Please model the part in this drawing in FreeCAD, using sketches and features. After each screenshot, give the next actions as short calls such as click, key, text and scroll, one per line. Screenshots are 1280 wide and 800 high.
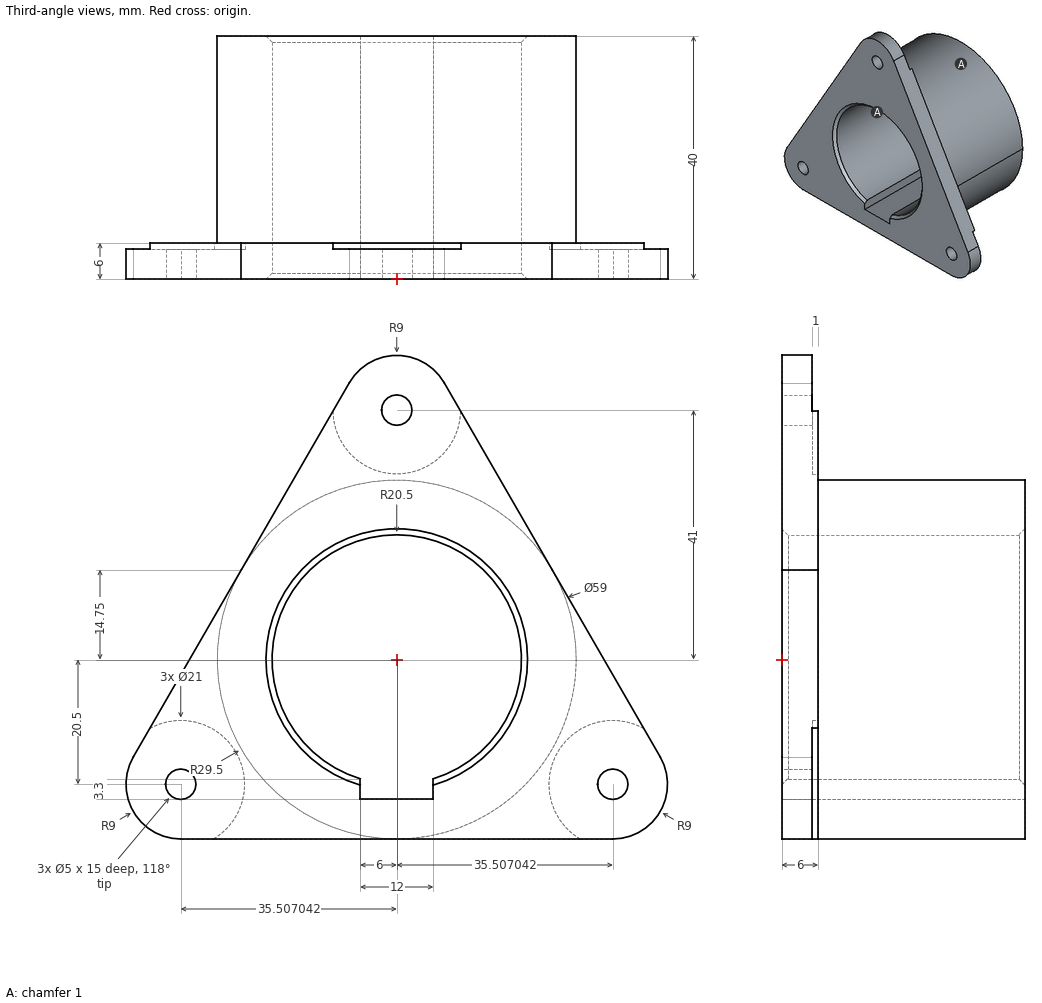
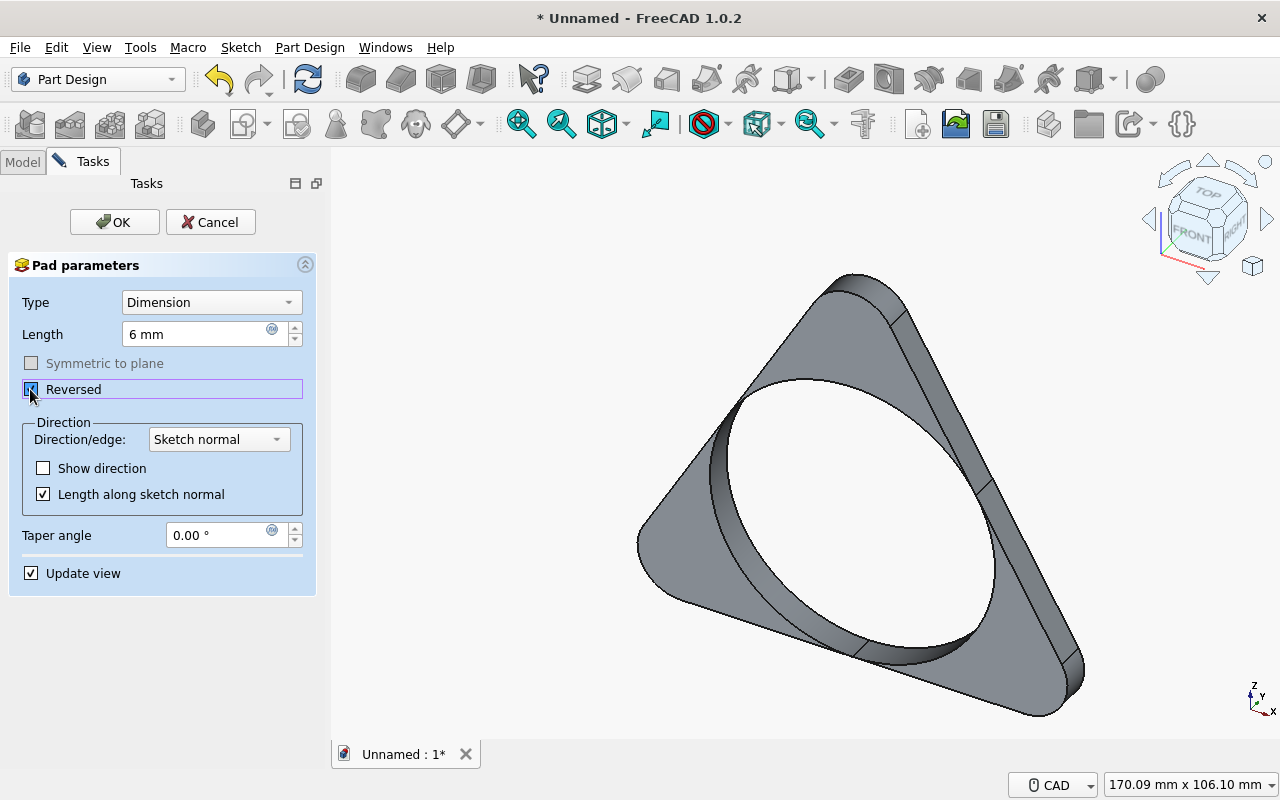
click(115, 222)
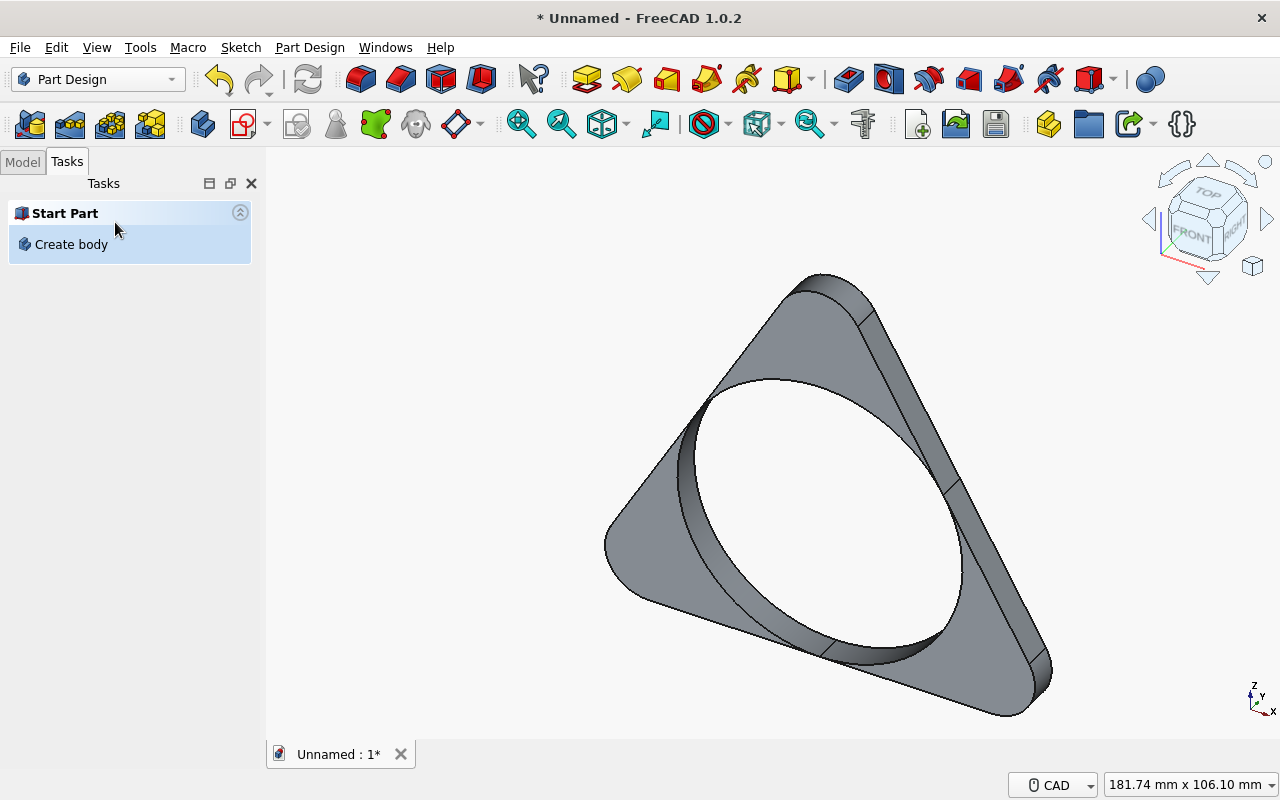
click(23, 161)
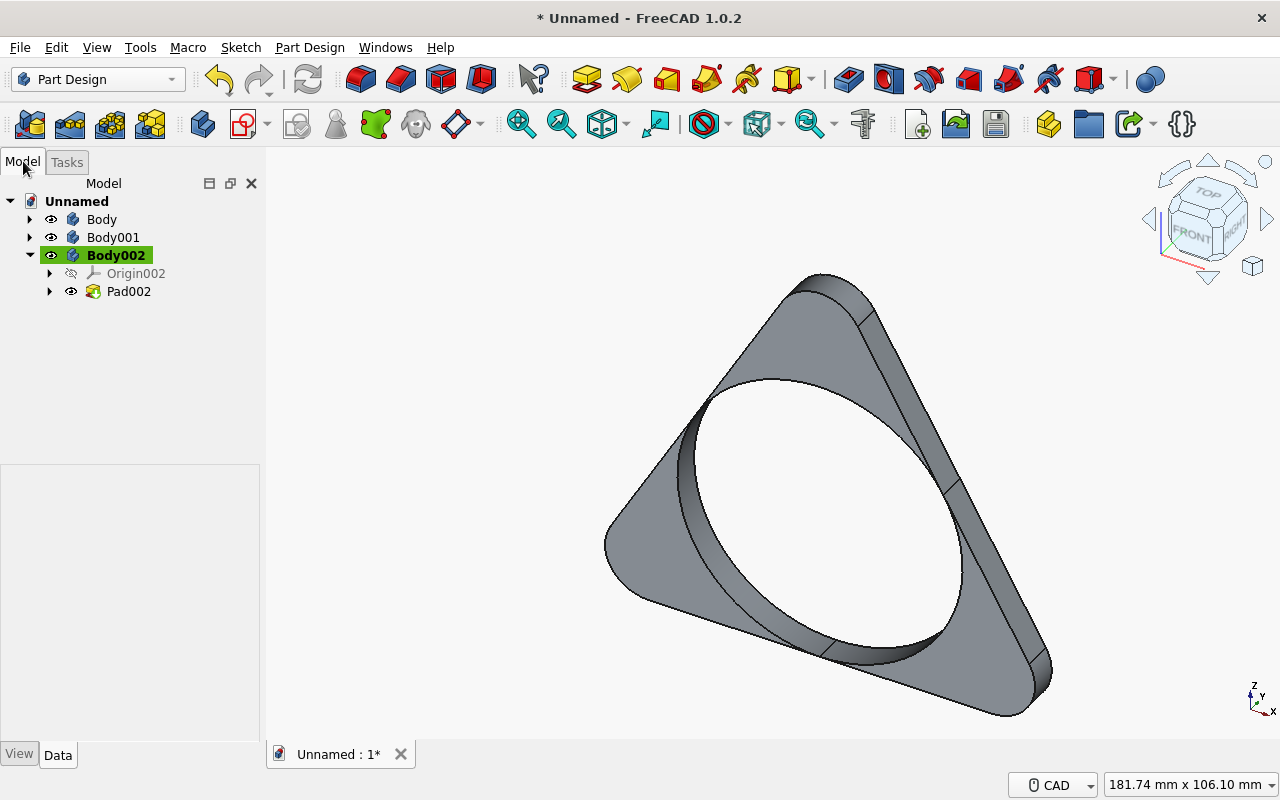
double_click(96, 219)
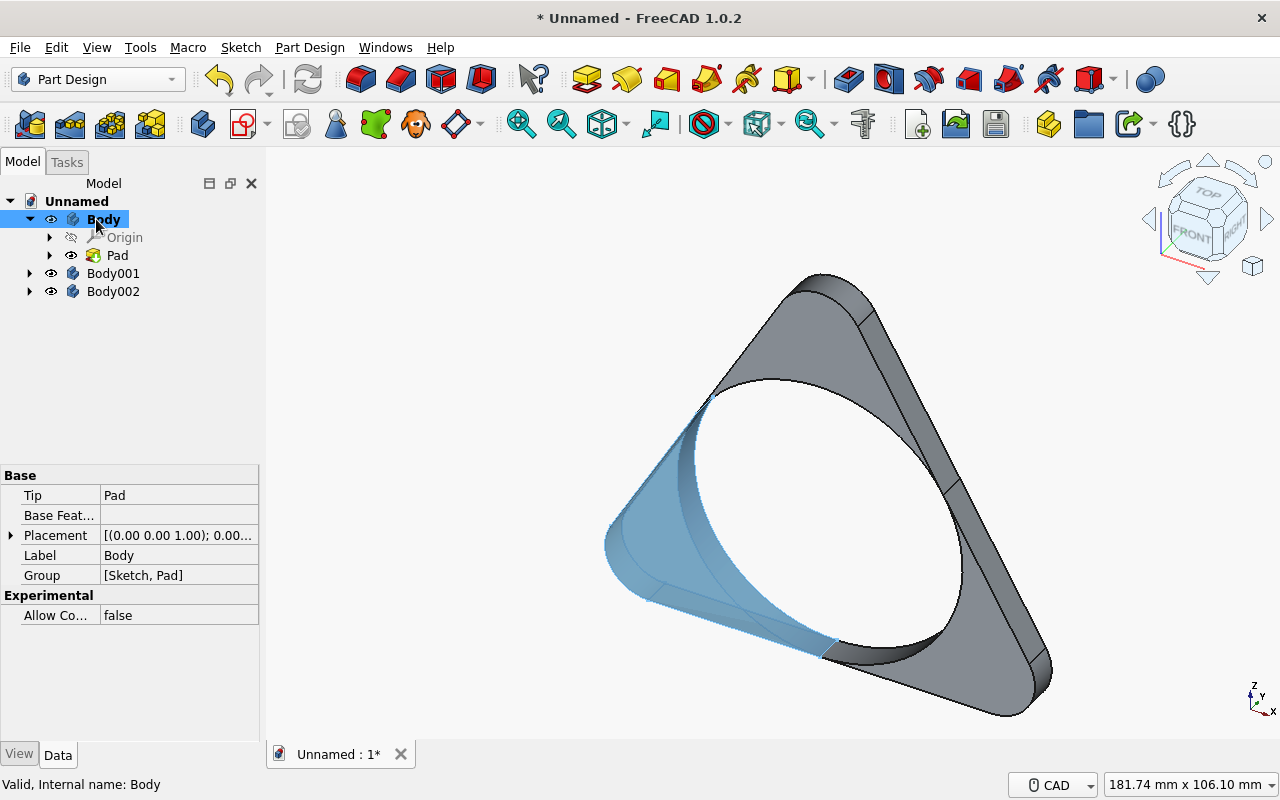
click(96, 219)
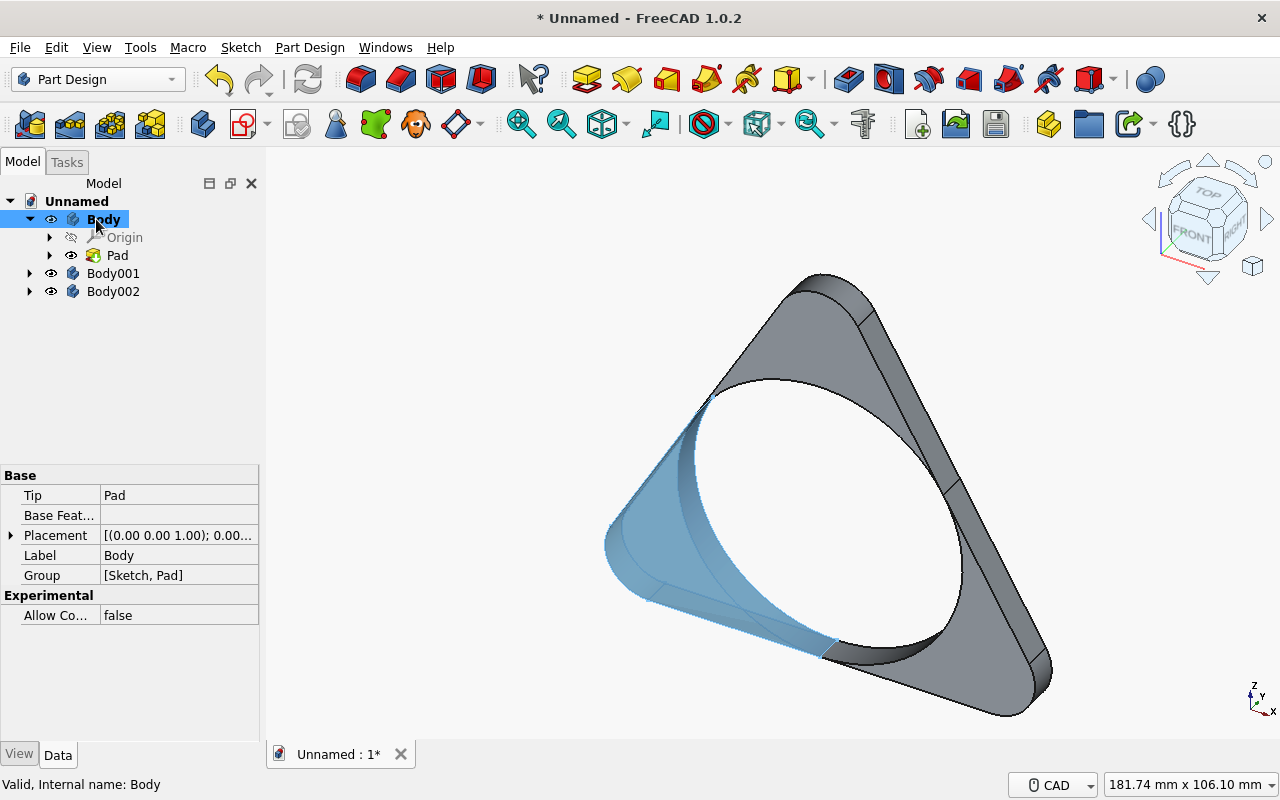
click(146, 615)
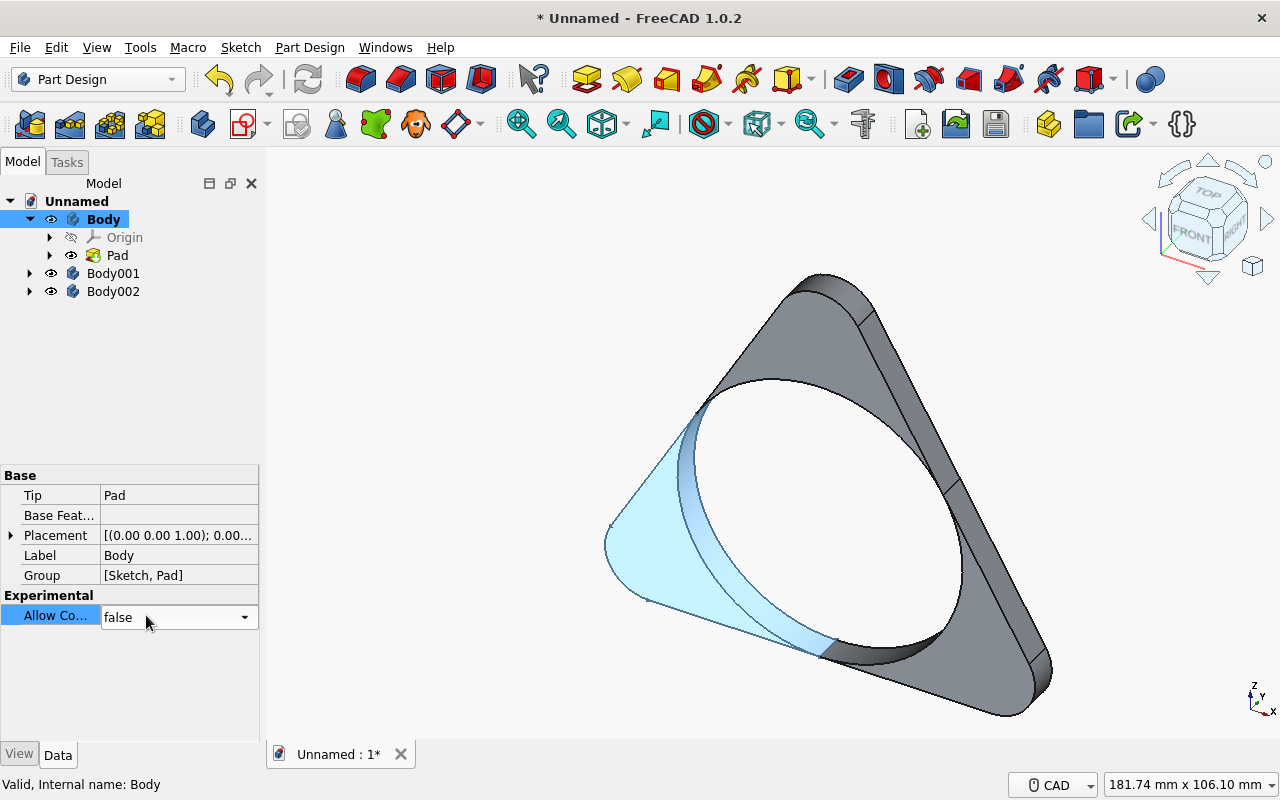
click(146, 615)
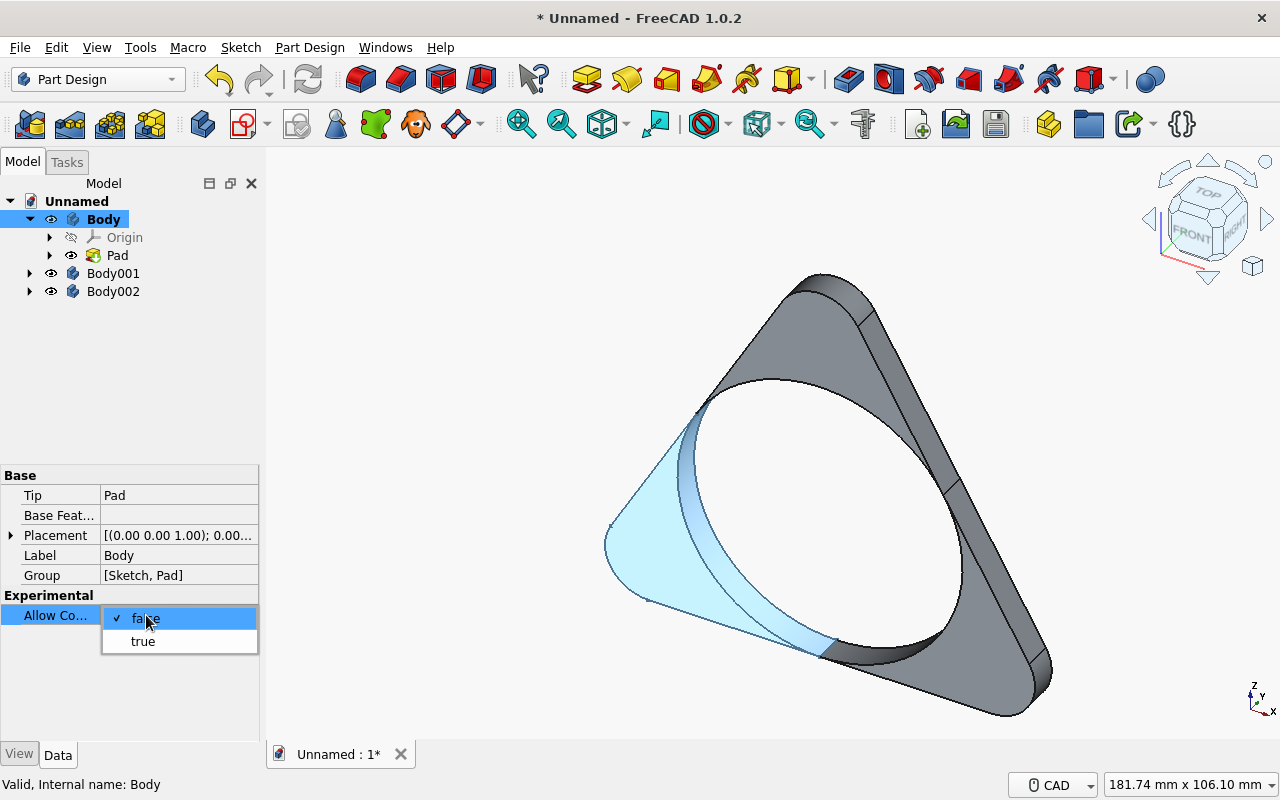
click(179, 642)
key(Return)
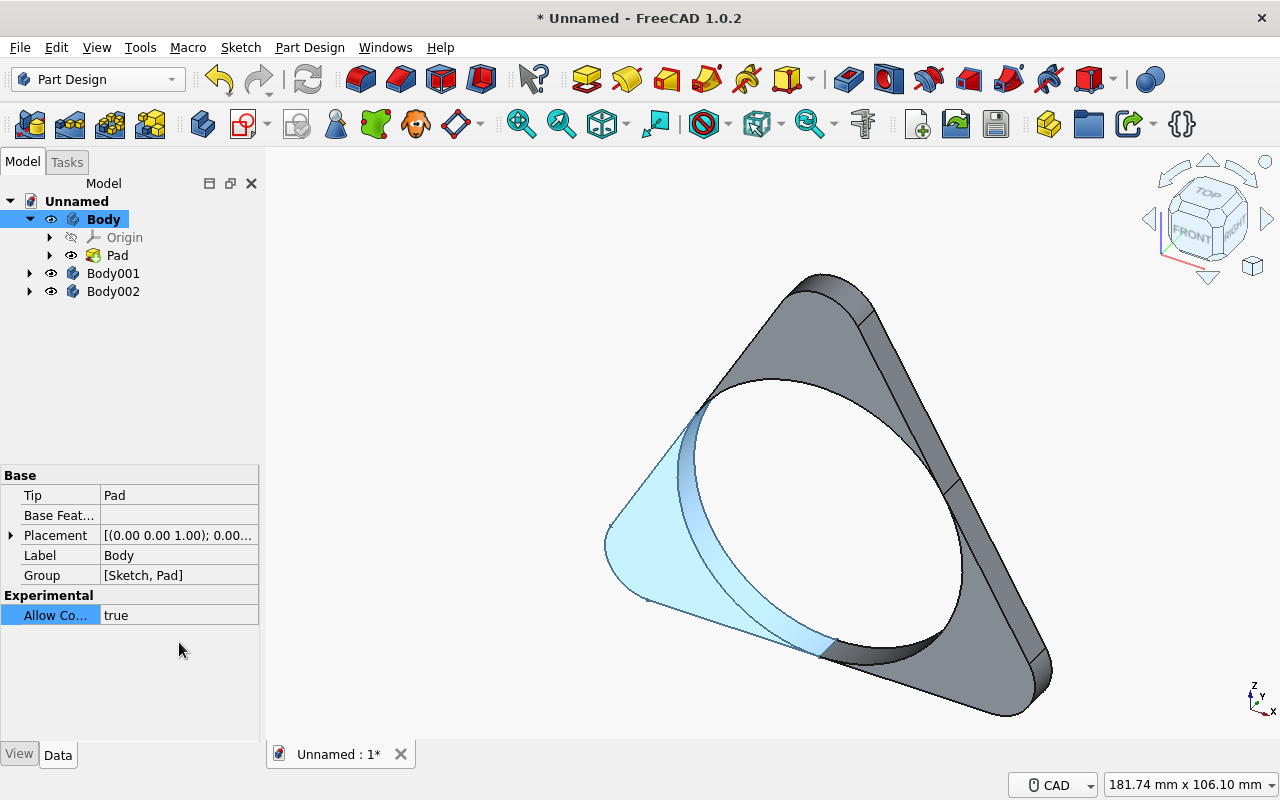
click(96, 273)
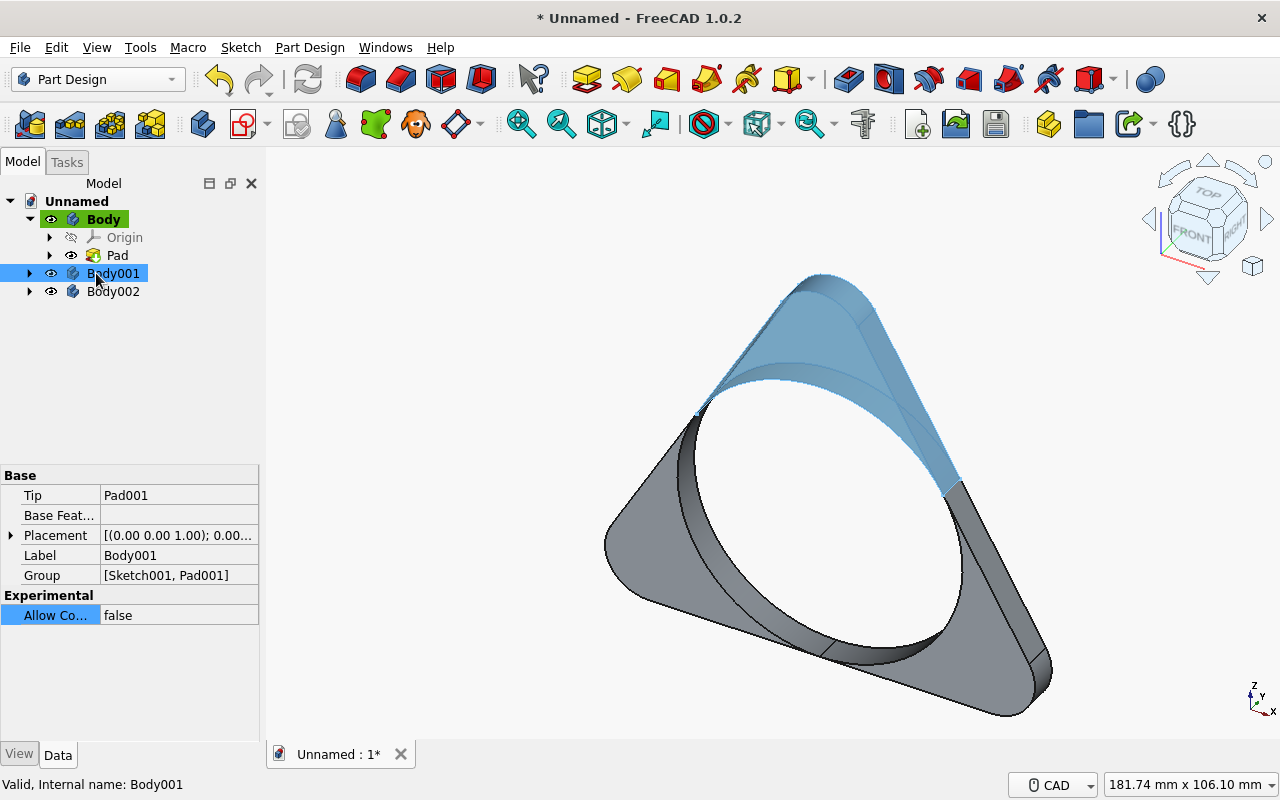
click(1152, 80)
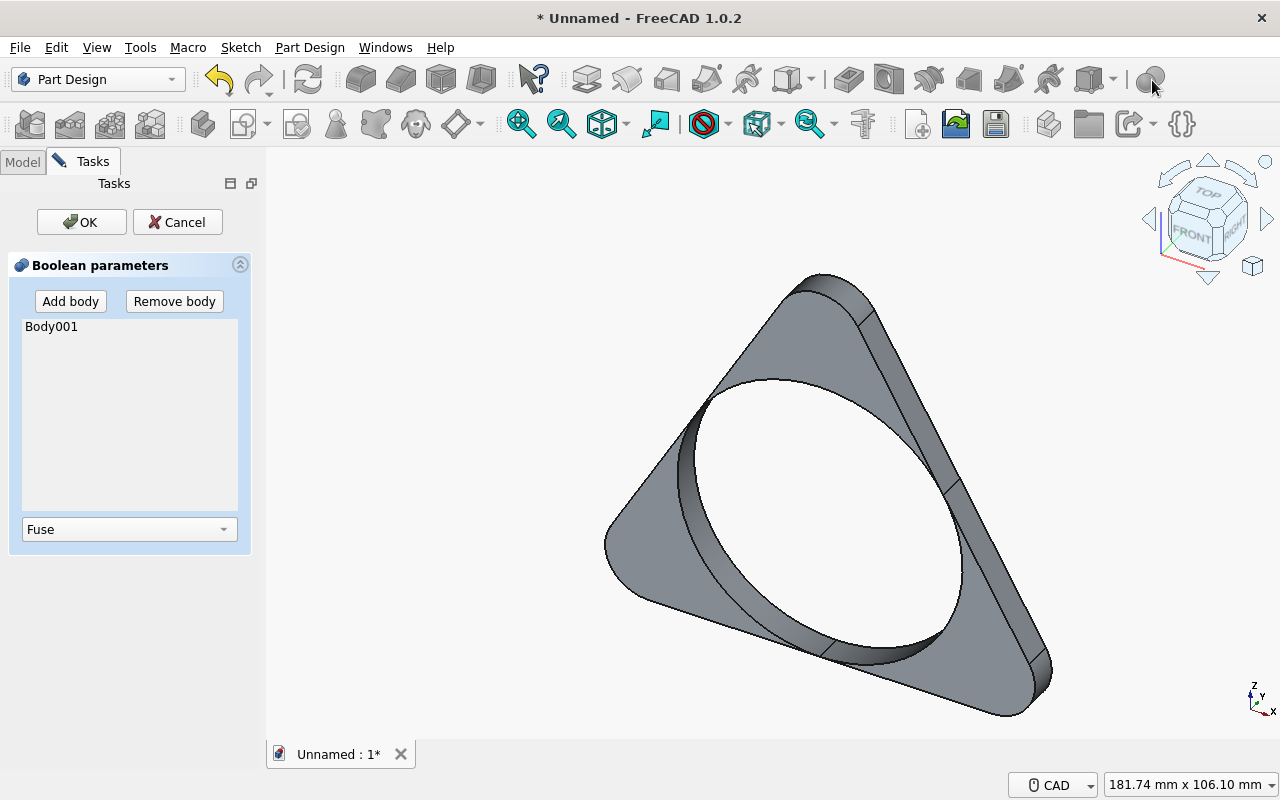
click(82, 222)